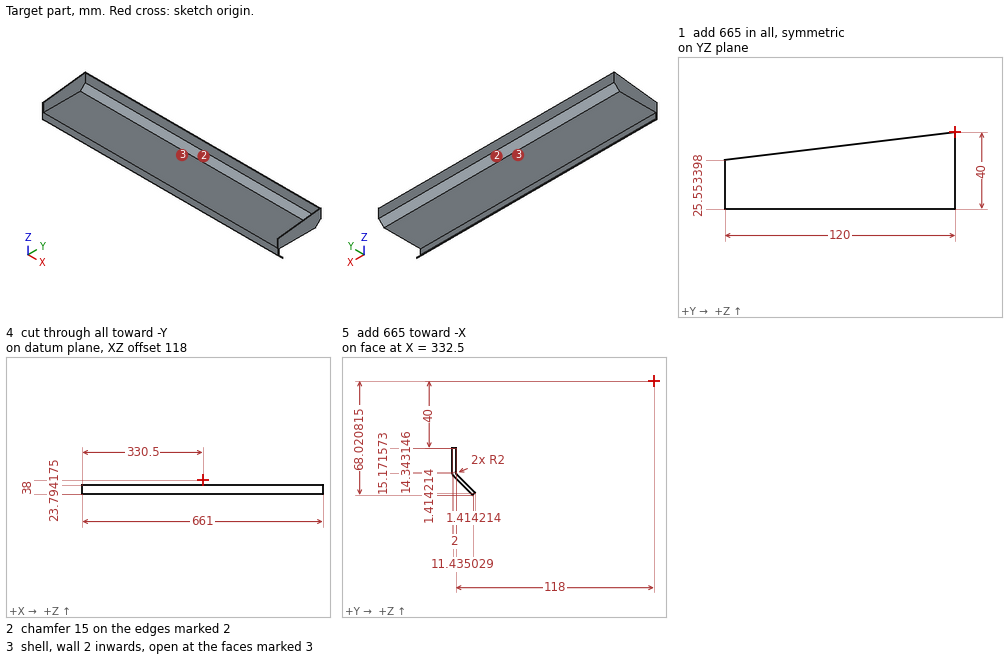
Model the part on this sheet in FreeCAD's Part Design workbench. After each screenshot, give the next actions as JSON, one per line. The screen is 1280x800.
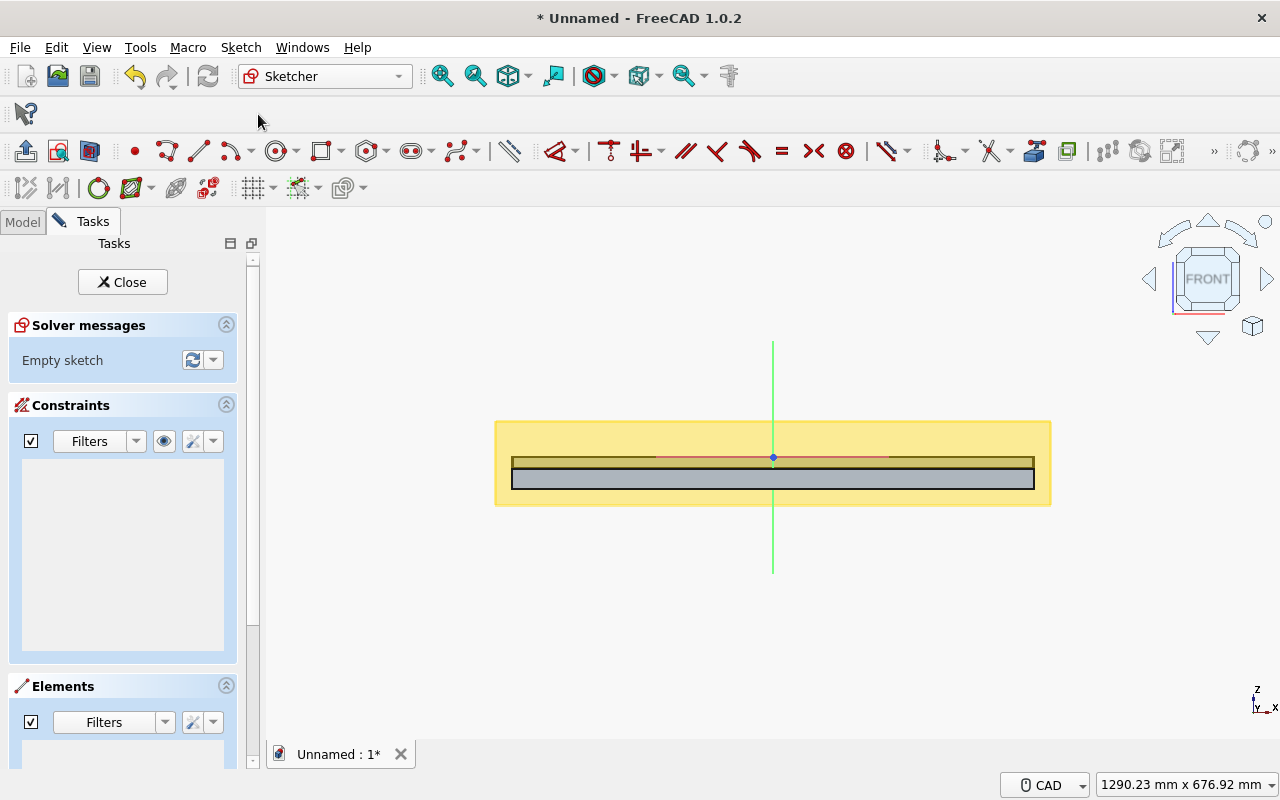
{"action": "left_click", "coordinate": [90, 152]}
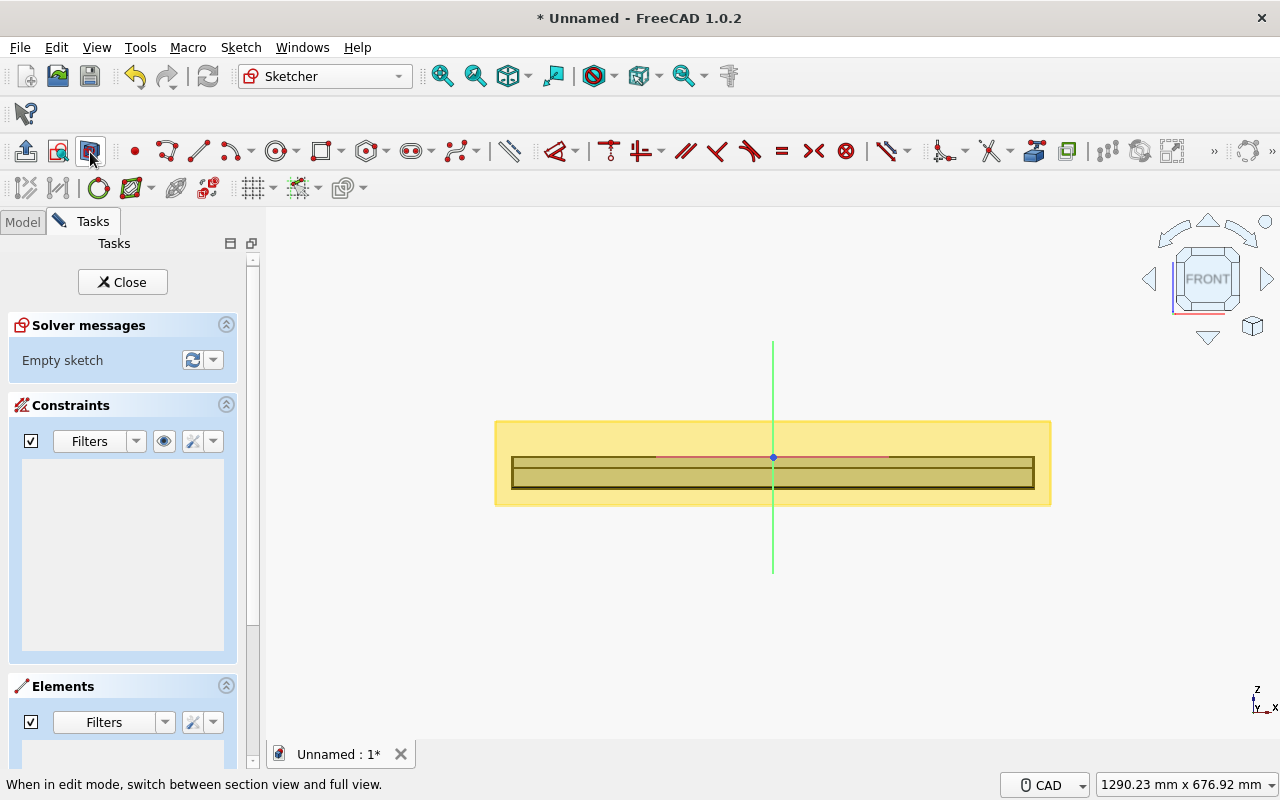
{"action": "key", "text": "g r"}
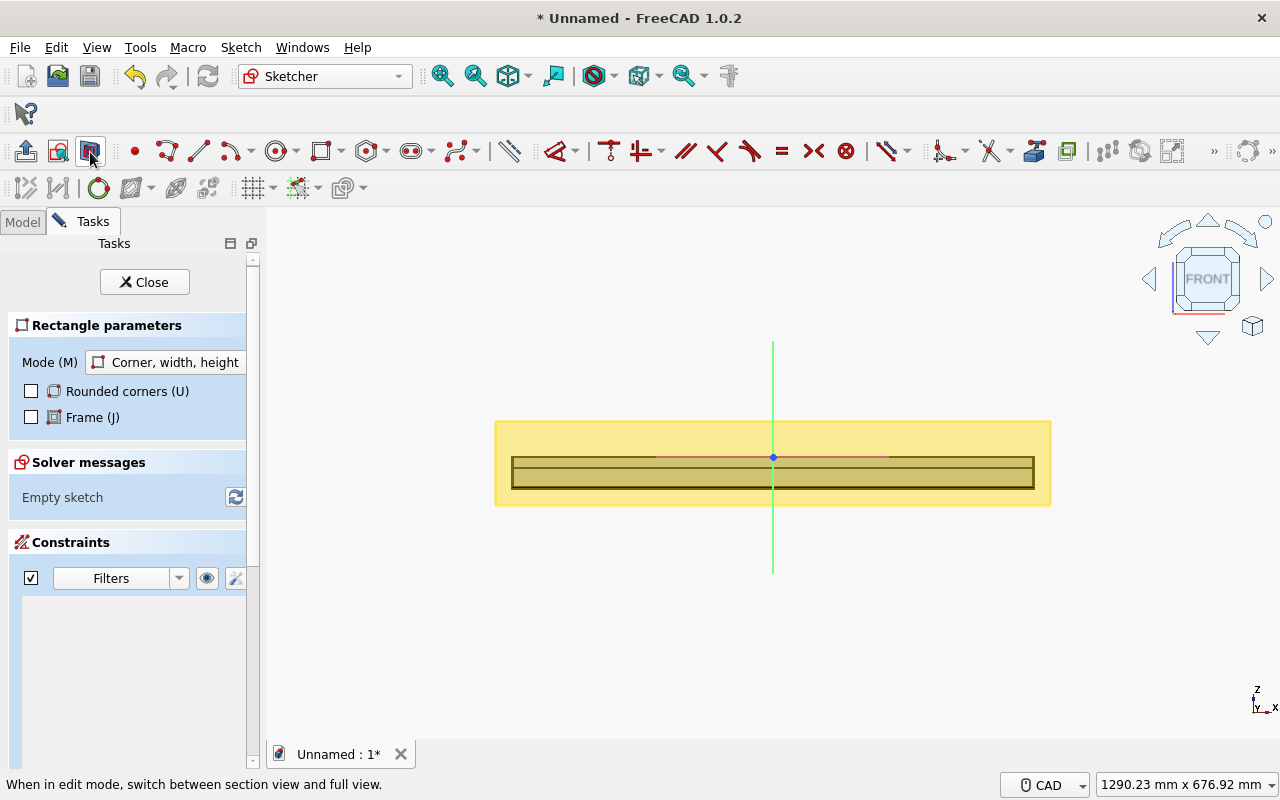
{"action": "scroll", "coordinate": [513, 468], "scroll_direction": "up", "scroll_amount": 2}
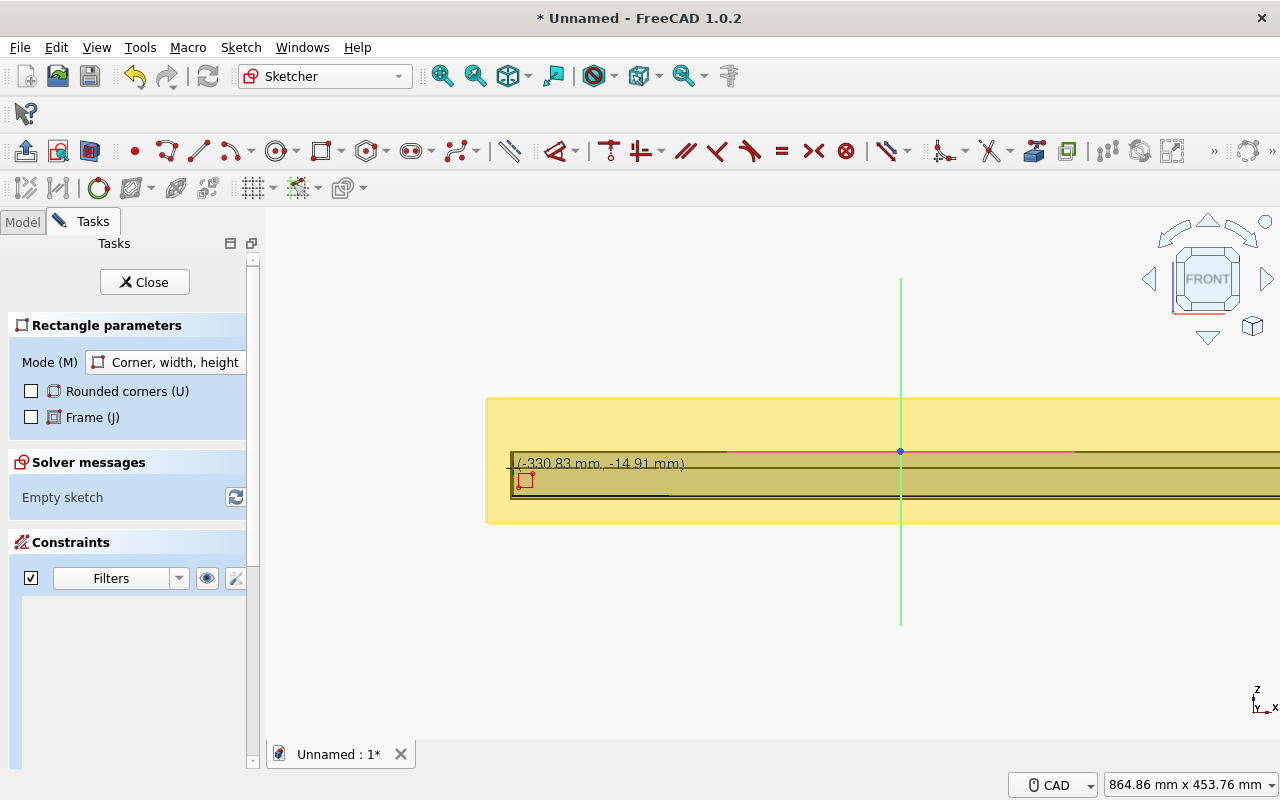
{"action": "left_click", "coordinate": [513, 468]}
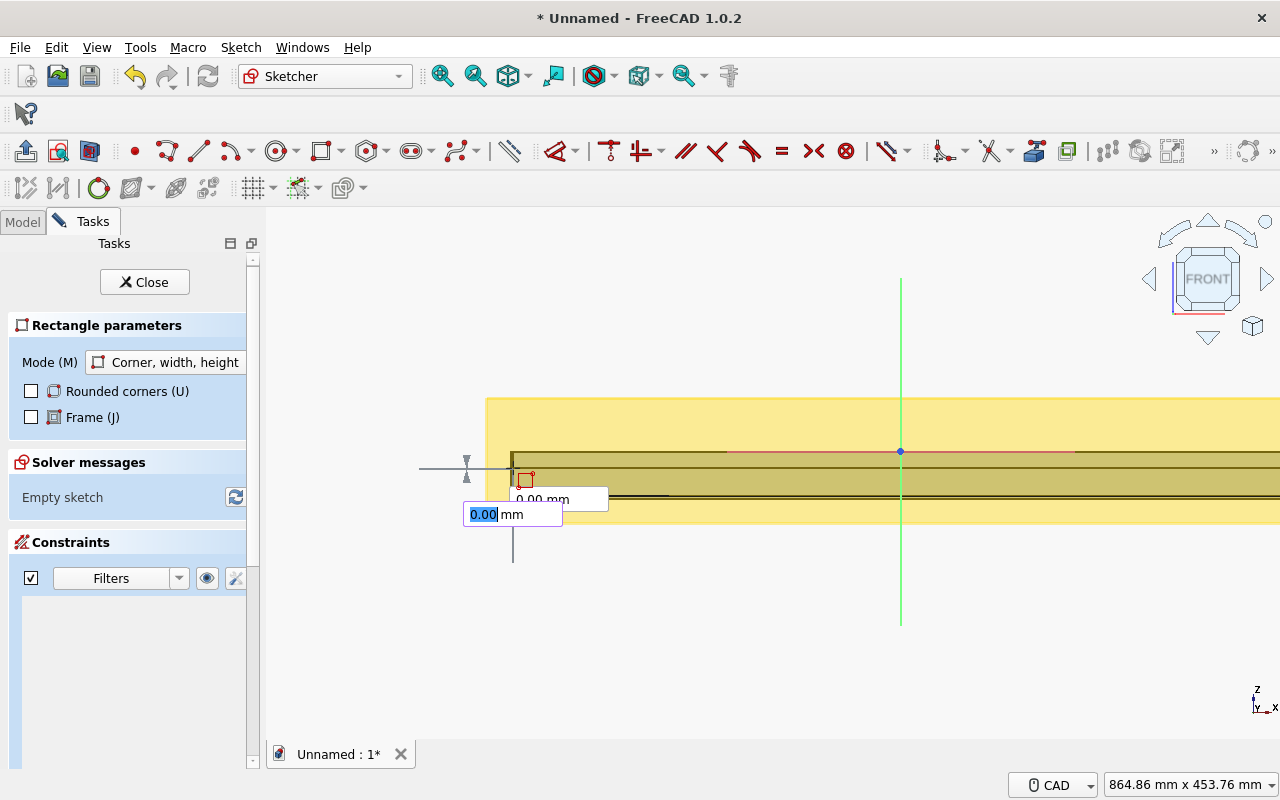
{"action": "scroll", "coordinate": [305, 471], "scroll_direction": "down", "scroll_amount": 2}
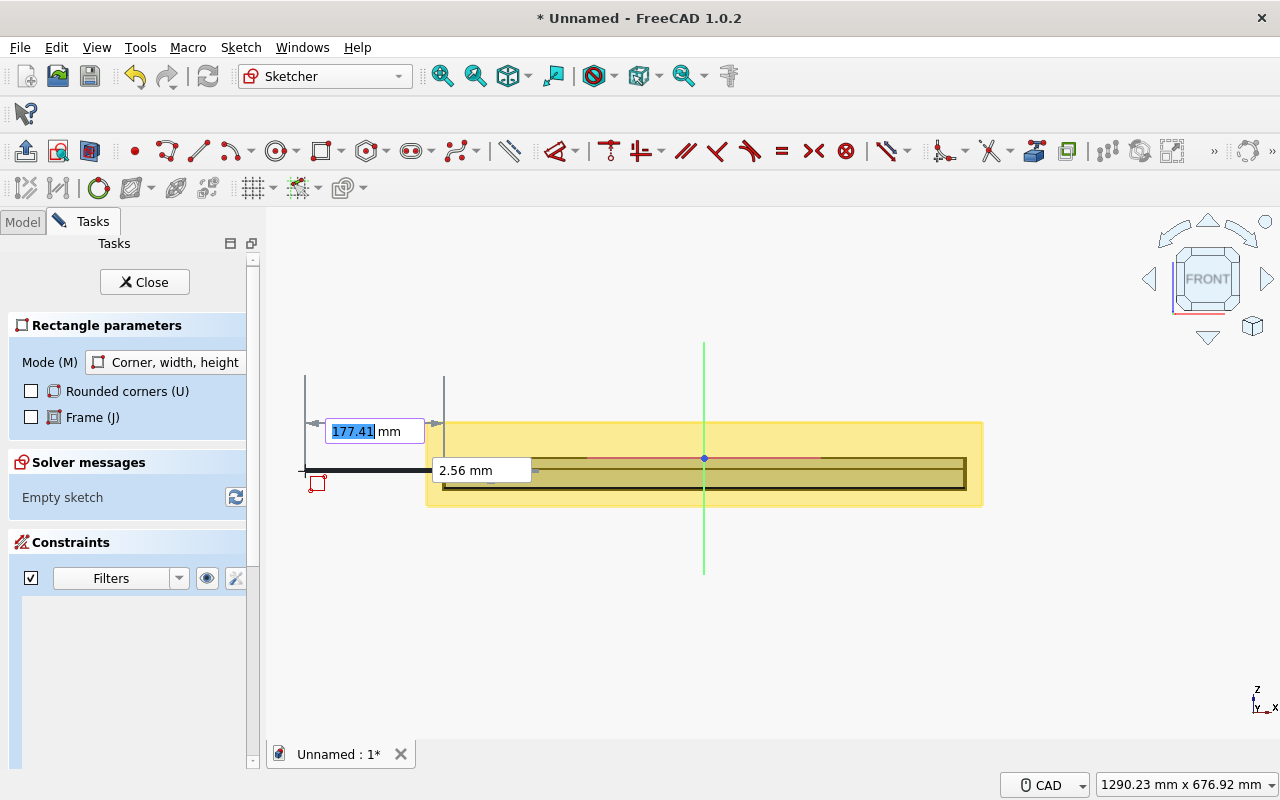
{"action": "left_click", "coordinate": [964, 488]}
{"action": "key", "text": "Escape"}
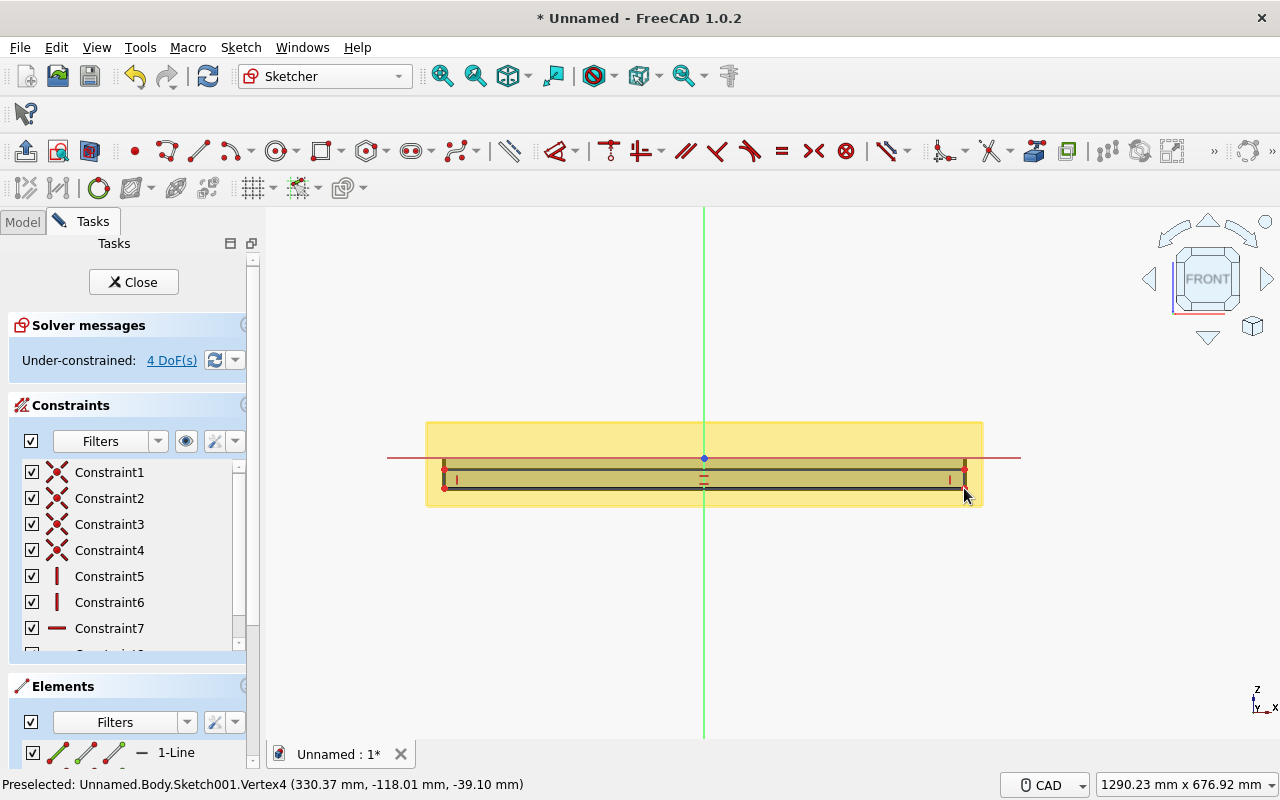
{"action": "key", "text": "d"}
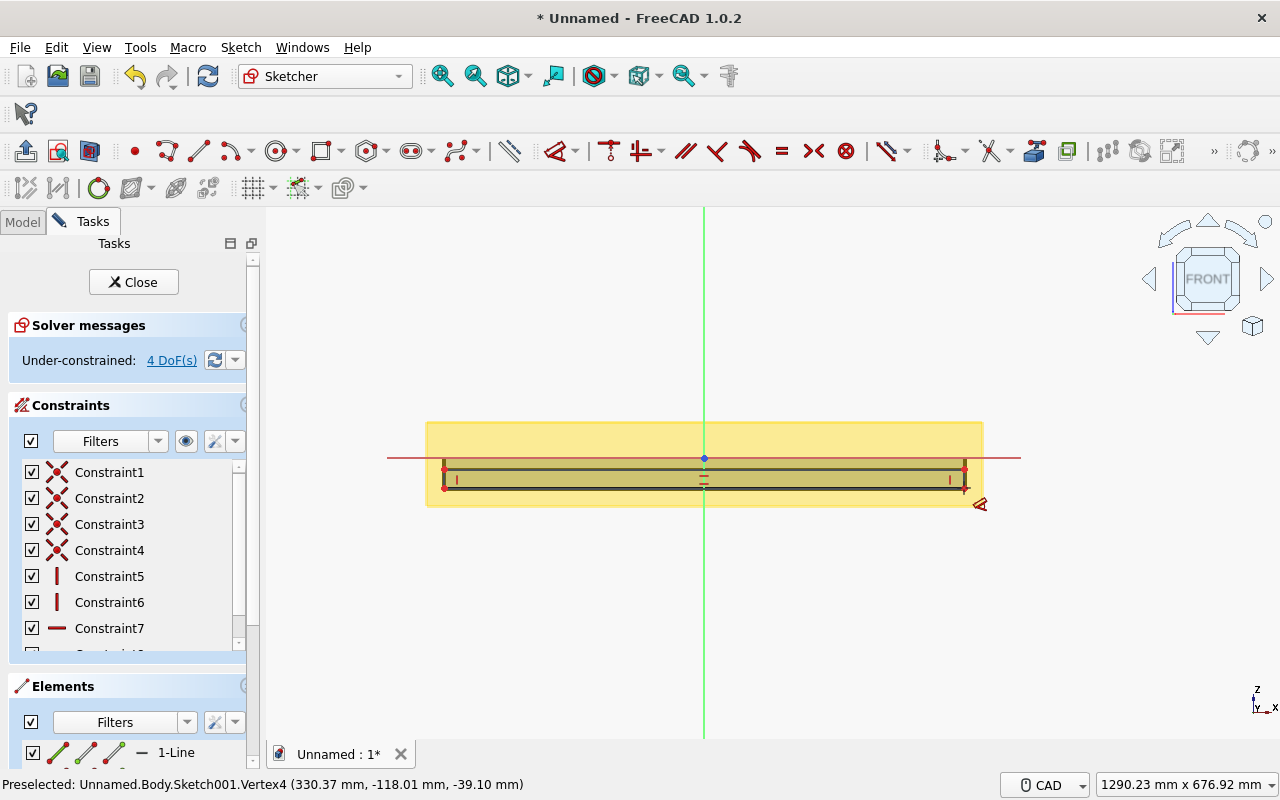
{"action": "left_click", "coordinate": [600, 489]}
{"action": "left_click", "coordinate": [585, 523]}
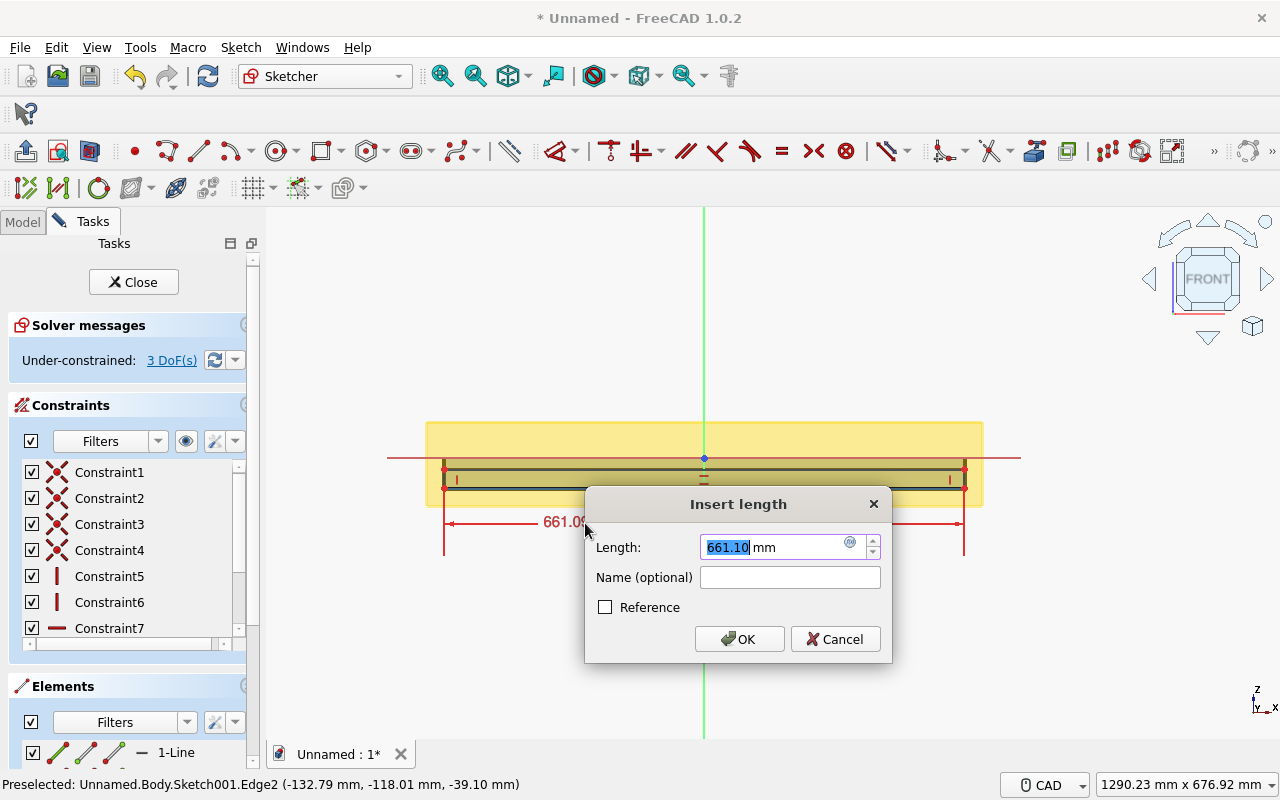
{"action": "type", "text": "661"}
{"action": "key", "text": "Return"}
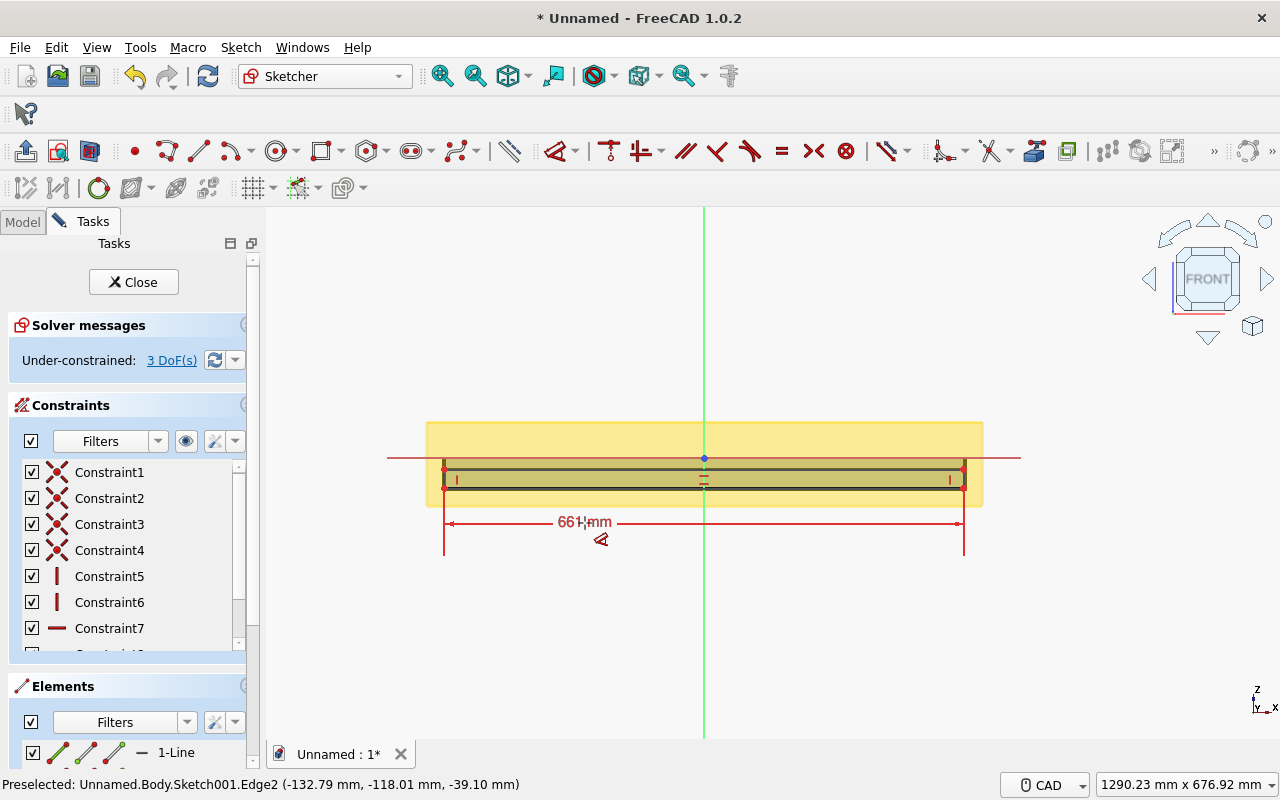
{"action": "scroll", "coordinate": [444, 489], "scroll_direction": "up", "scroll_amount": 2}